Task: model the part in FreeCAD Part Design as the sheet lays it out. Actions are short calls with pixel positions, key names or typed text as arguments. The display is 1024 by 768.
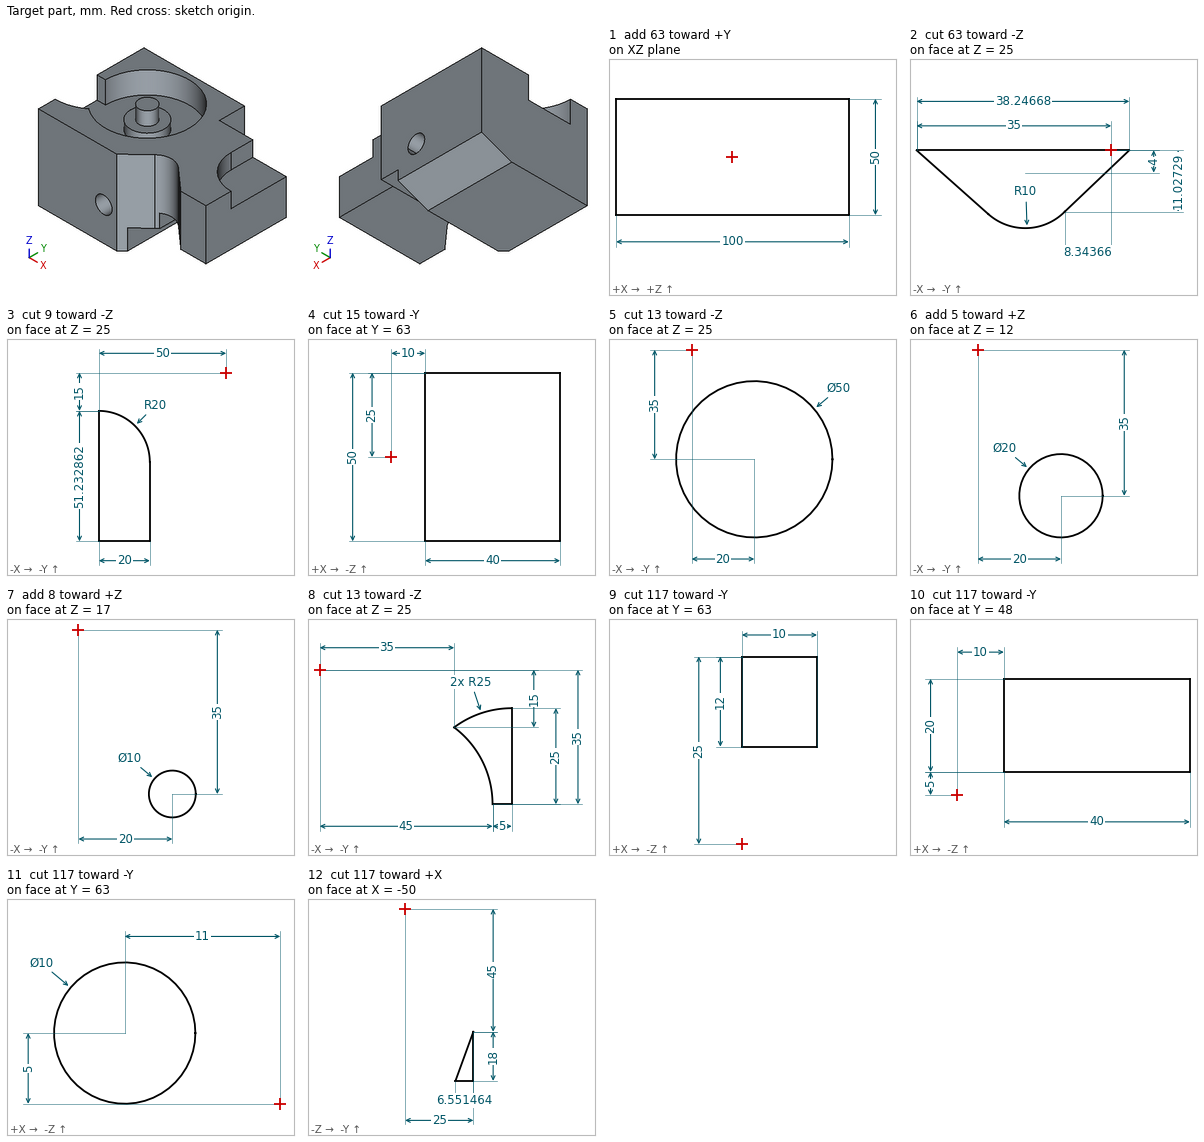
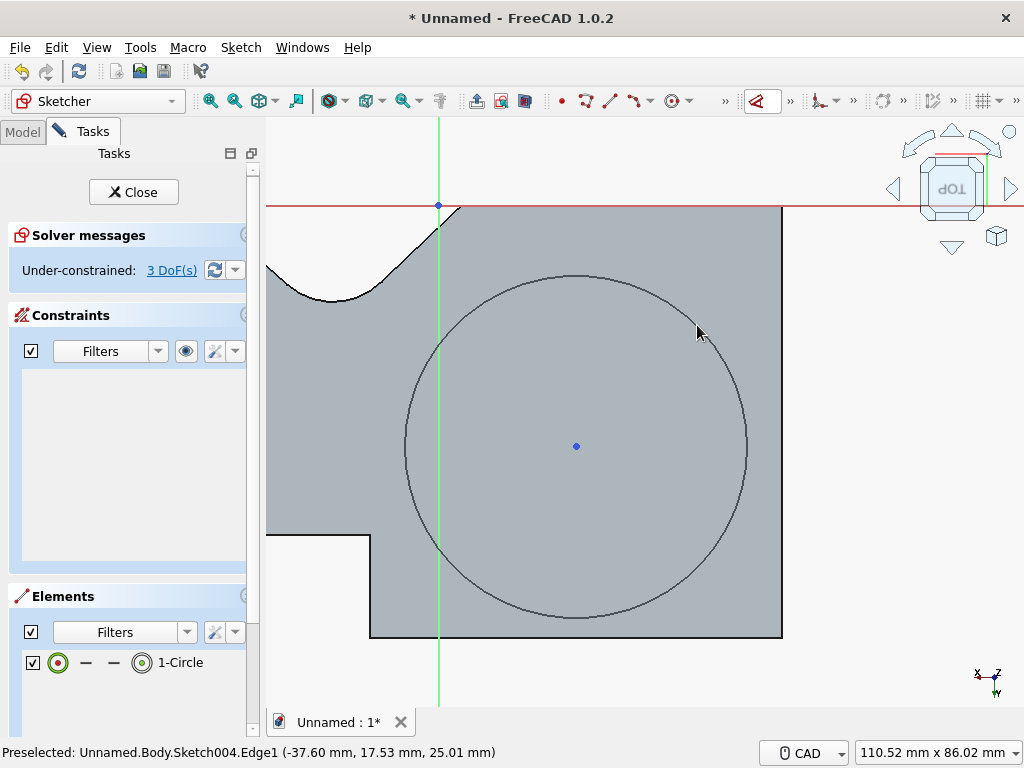
click(697, 326)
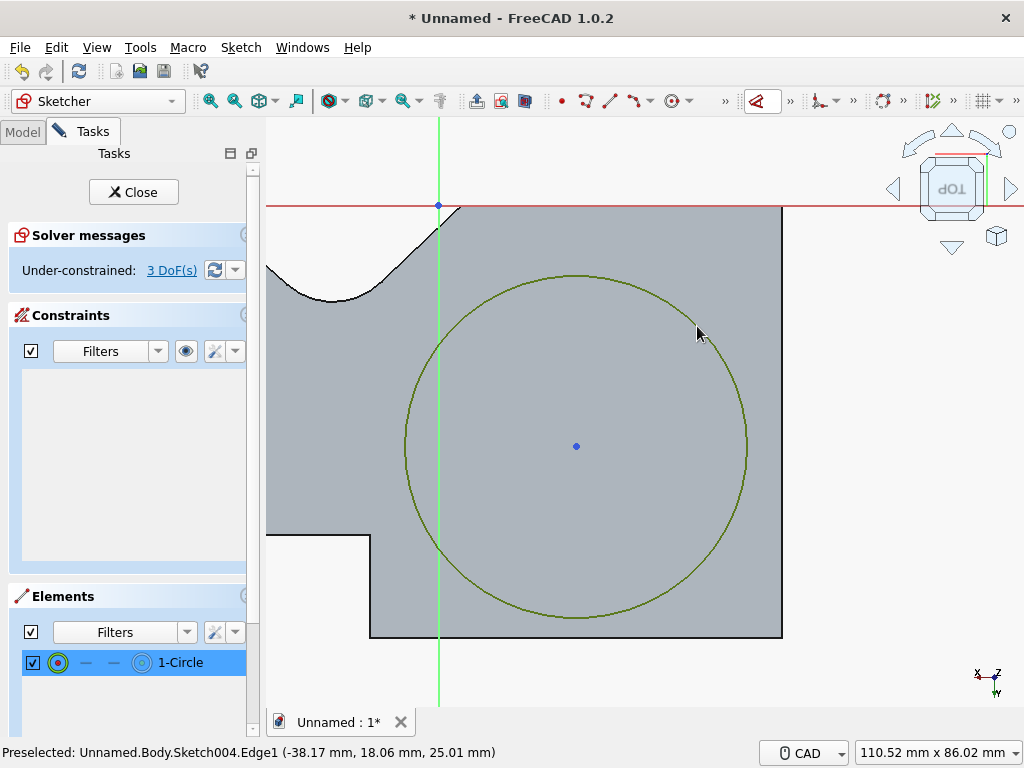
key(k)
key(o)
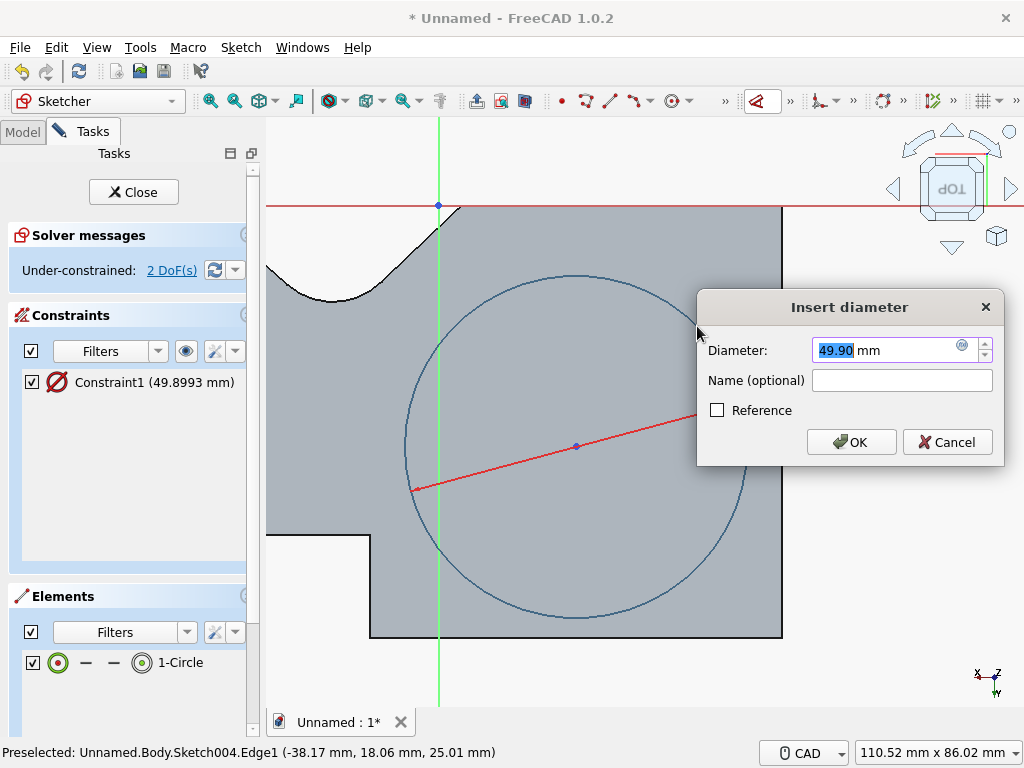
text(50)
key(Return)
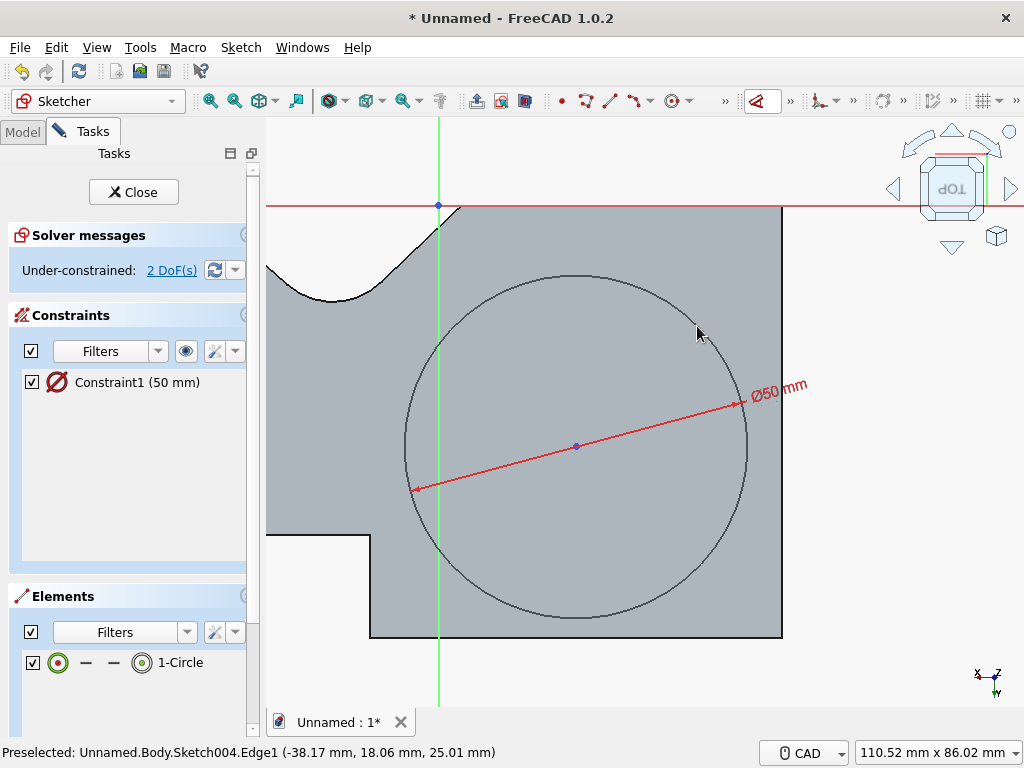
click(576, 447)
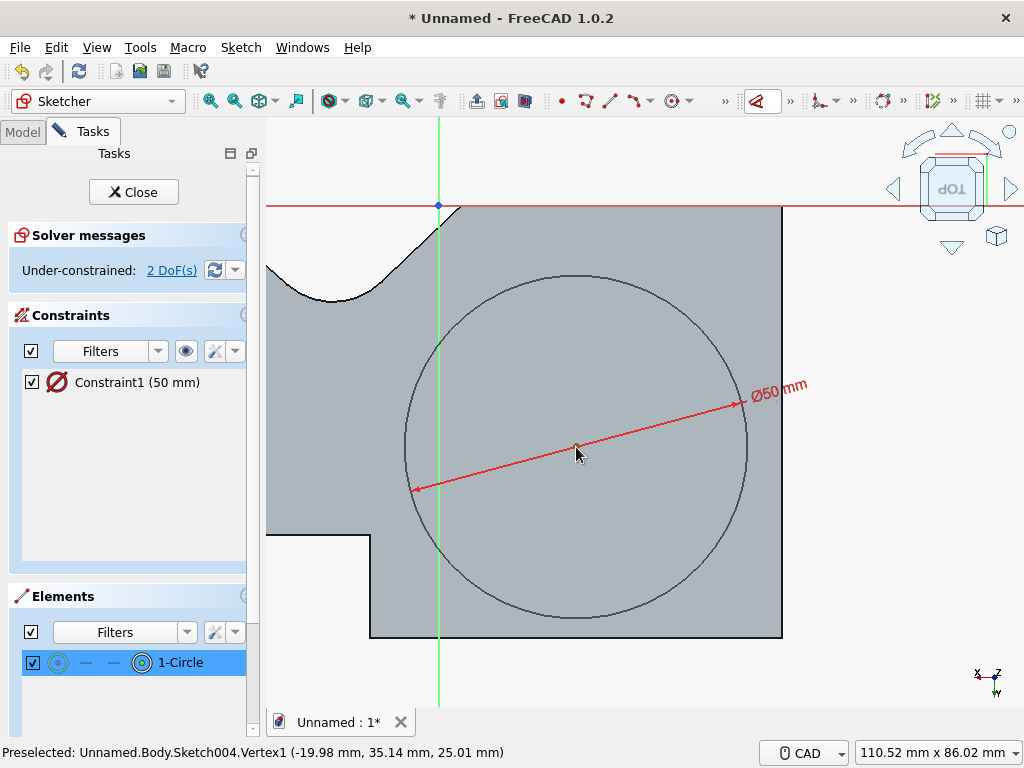
key(l)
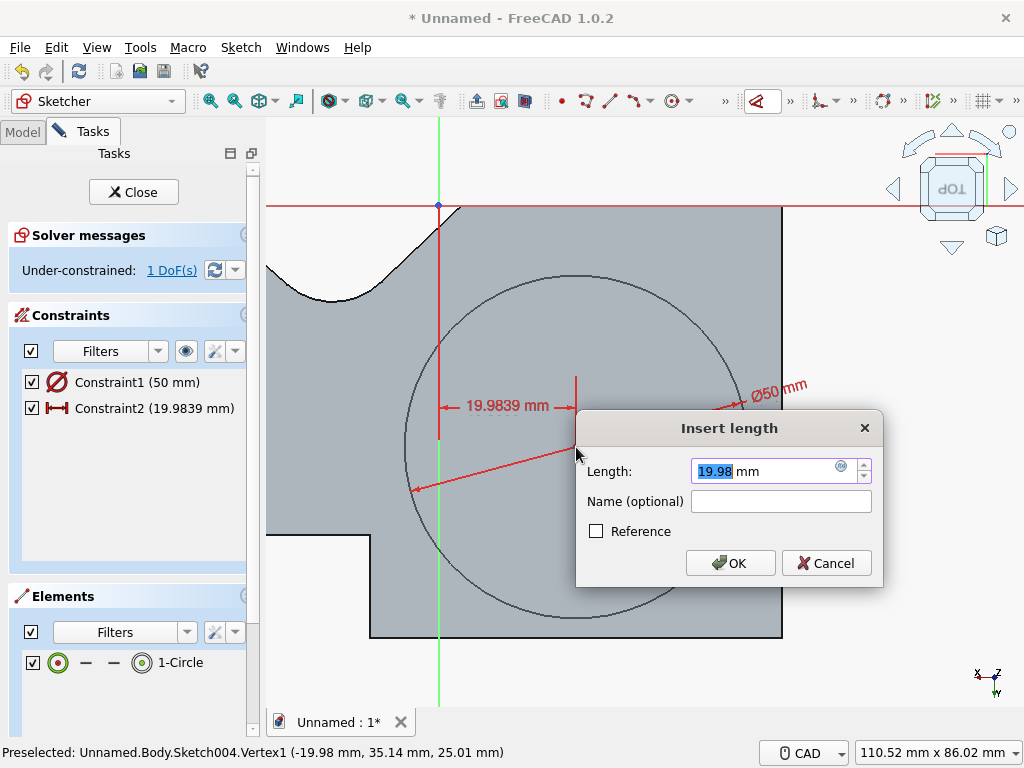
text(20)
key(Return)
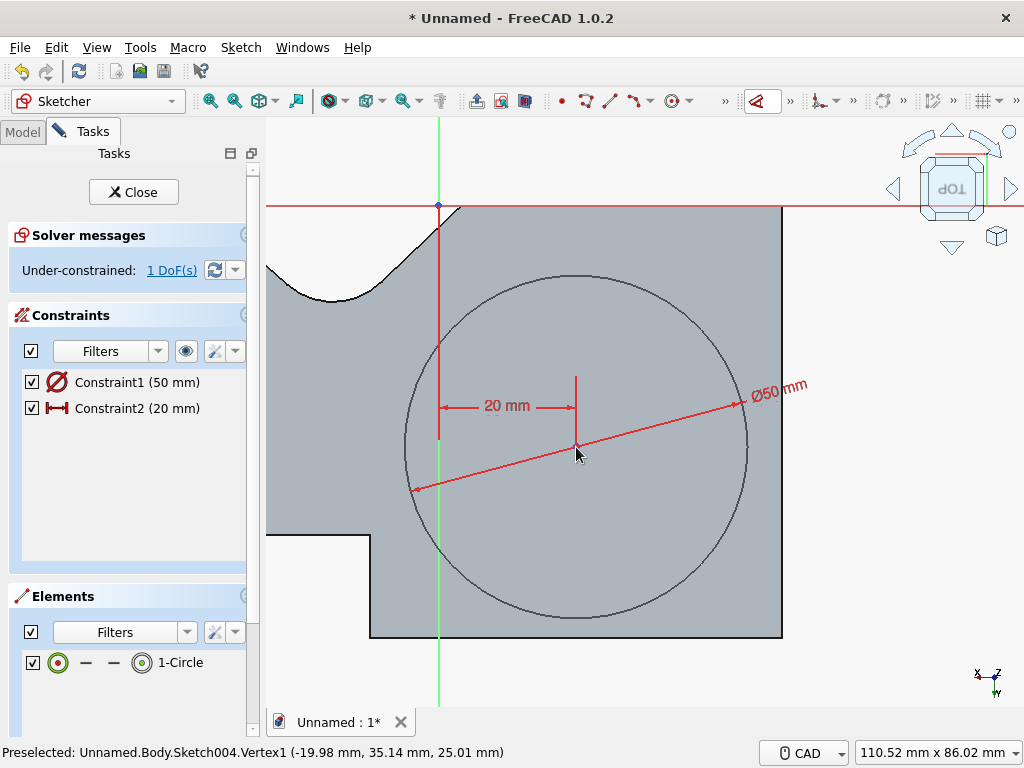
click(576, 447)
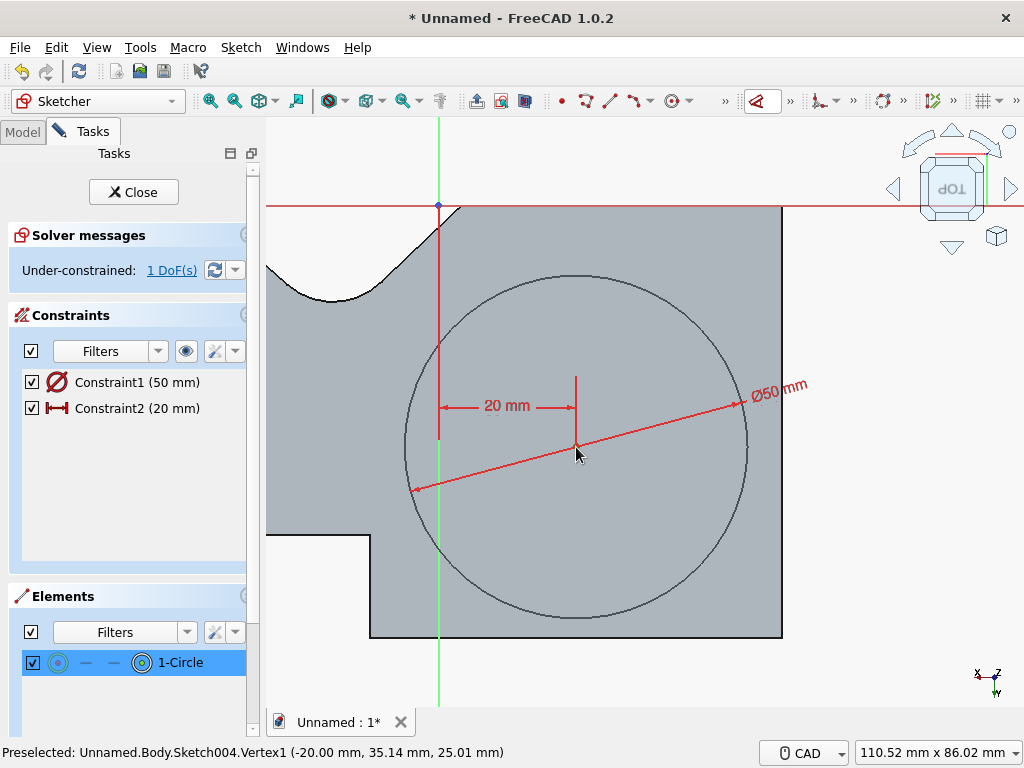
click(776, 102)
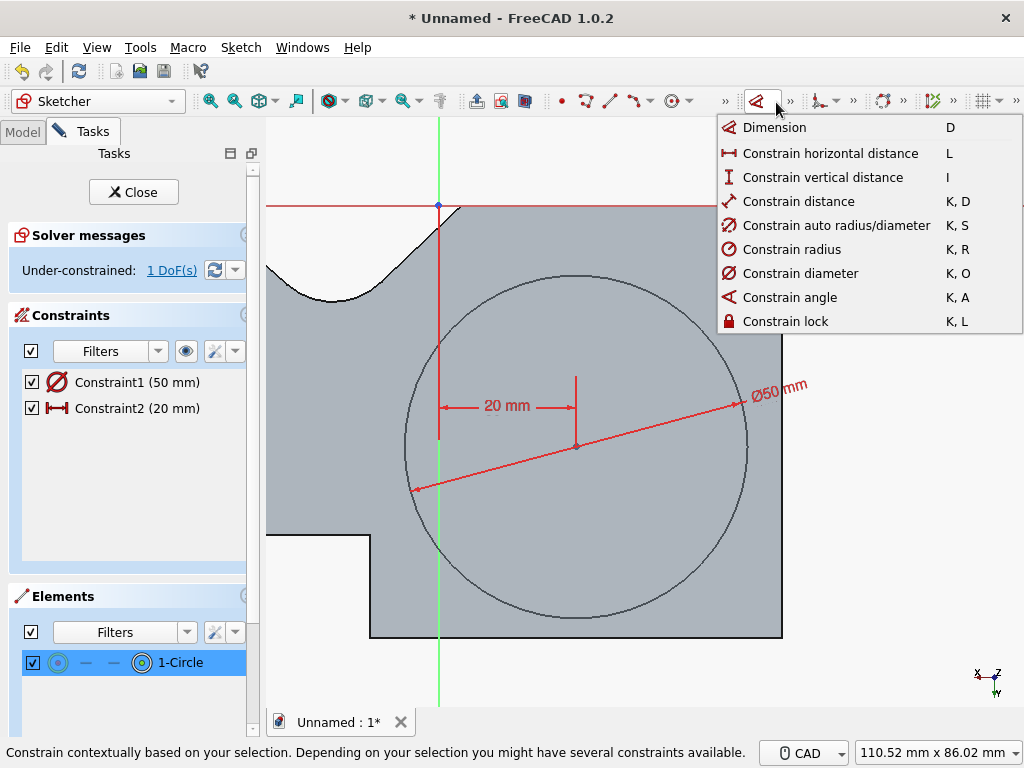
click(870, 177)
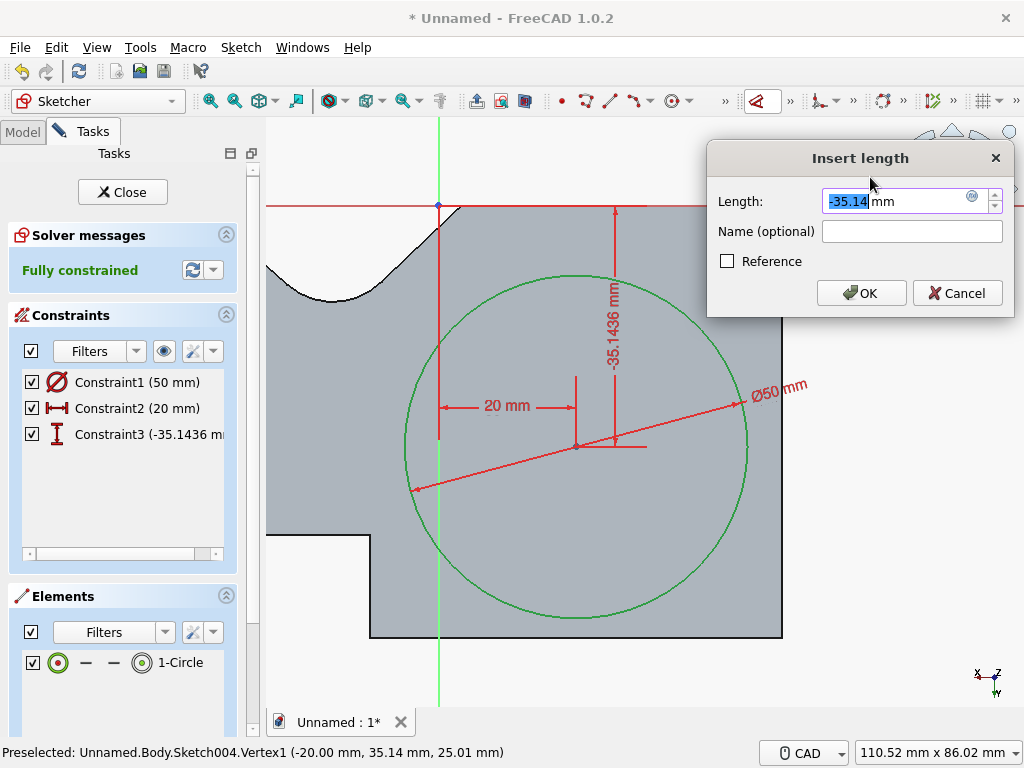
text(-35)
key(Return)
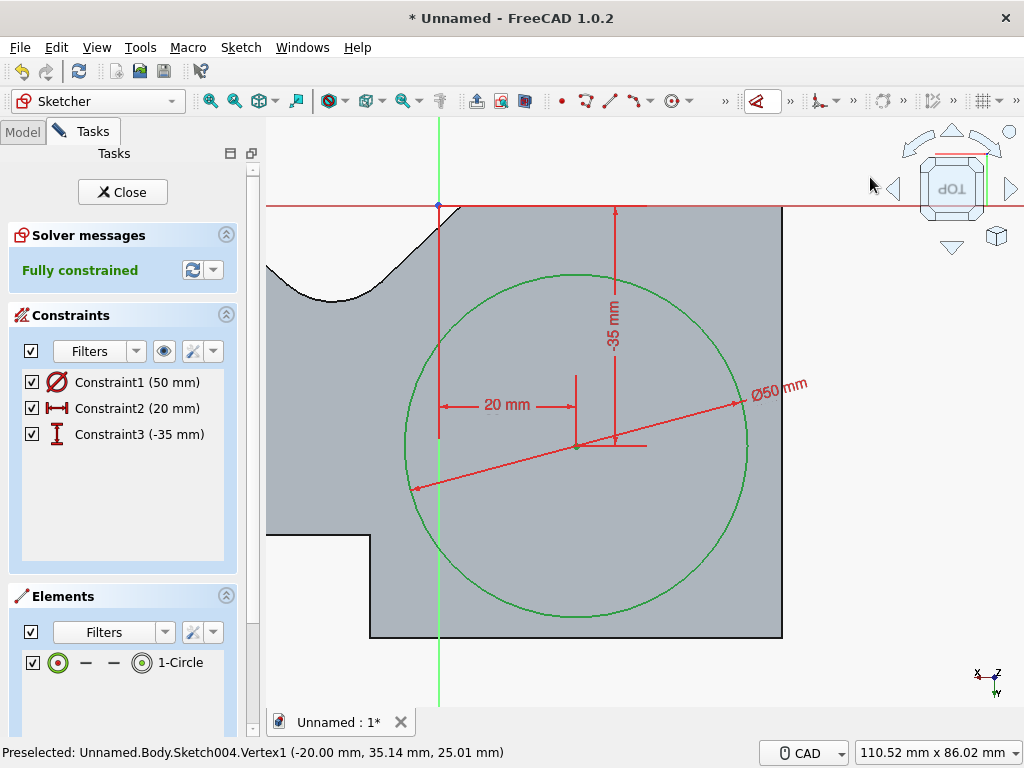
click(123, 192)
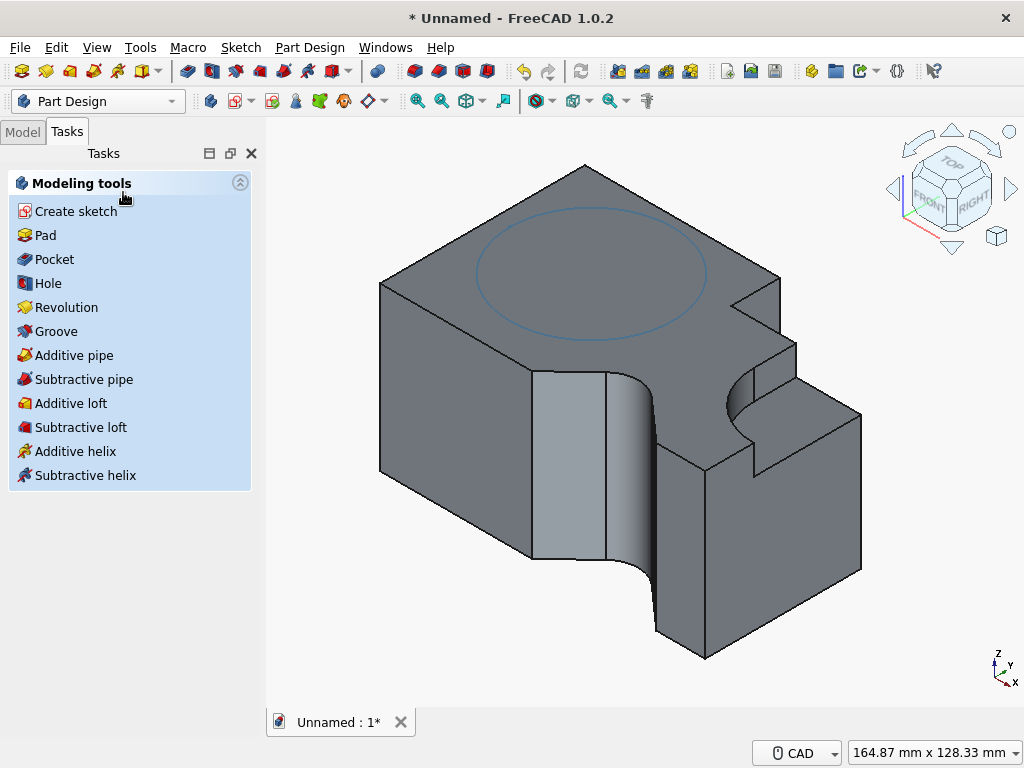
click(188, 72)